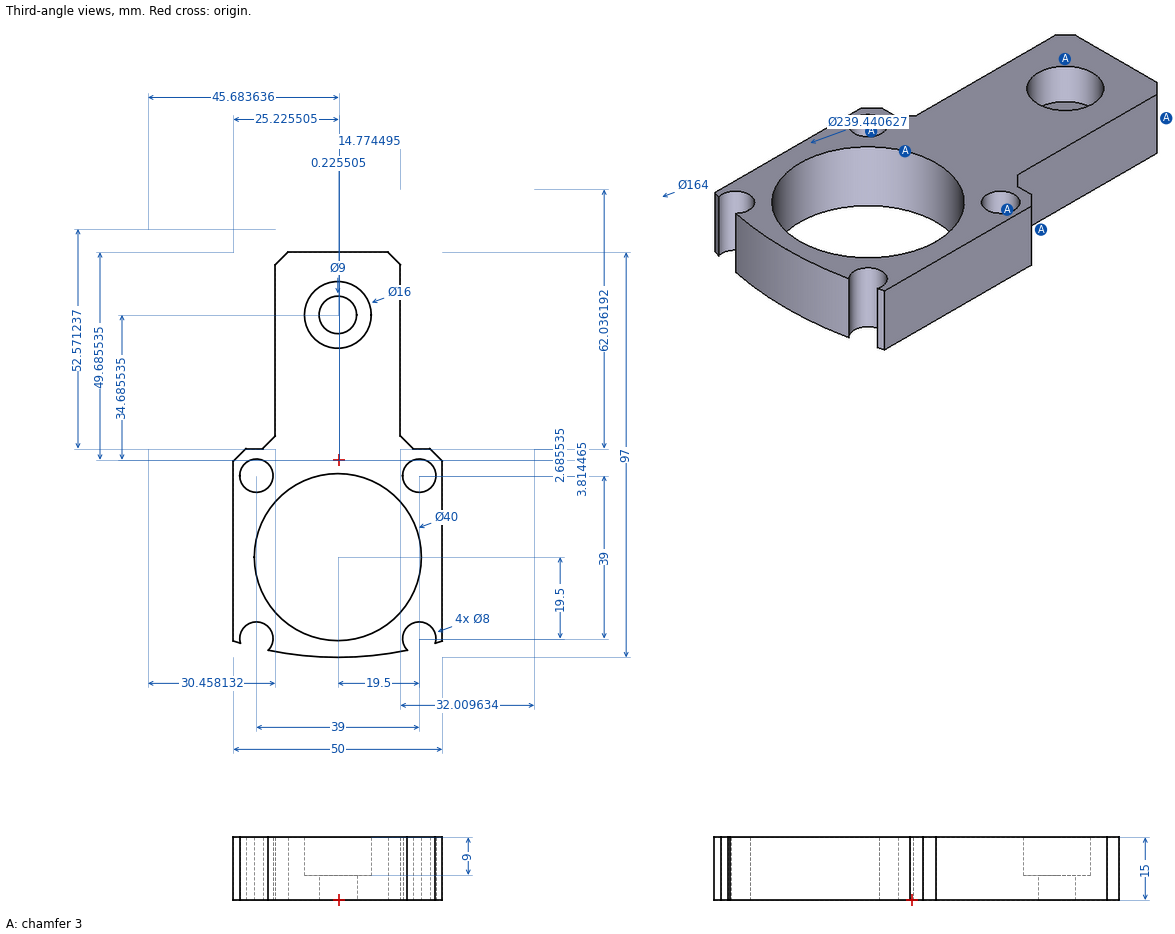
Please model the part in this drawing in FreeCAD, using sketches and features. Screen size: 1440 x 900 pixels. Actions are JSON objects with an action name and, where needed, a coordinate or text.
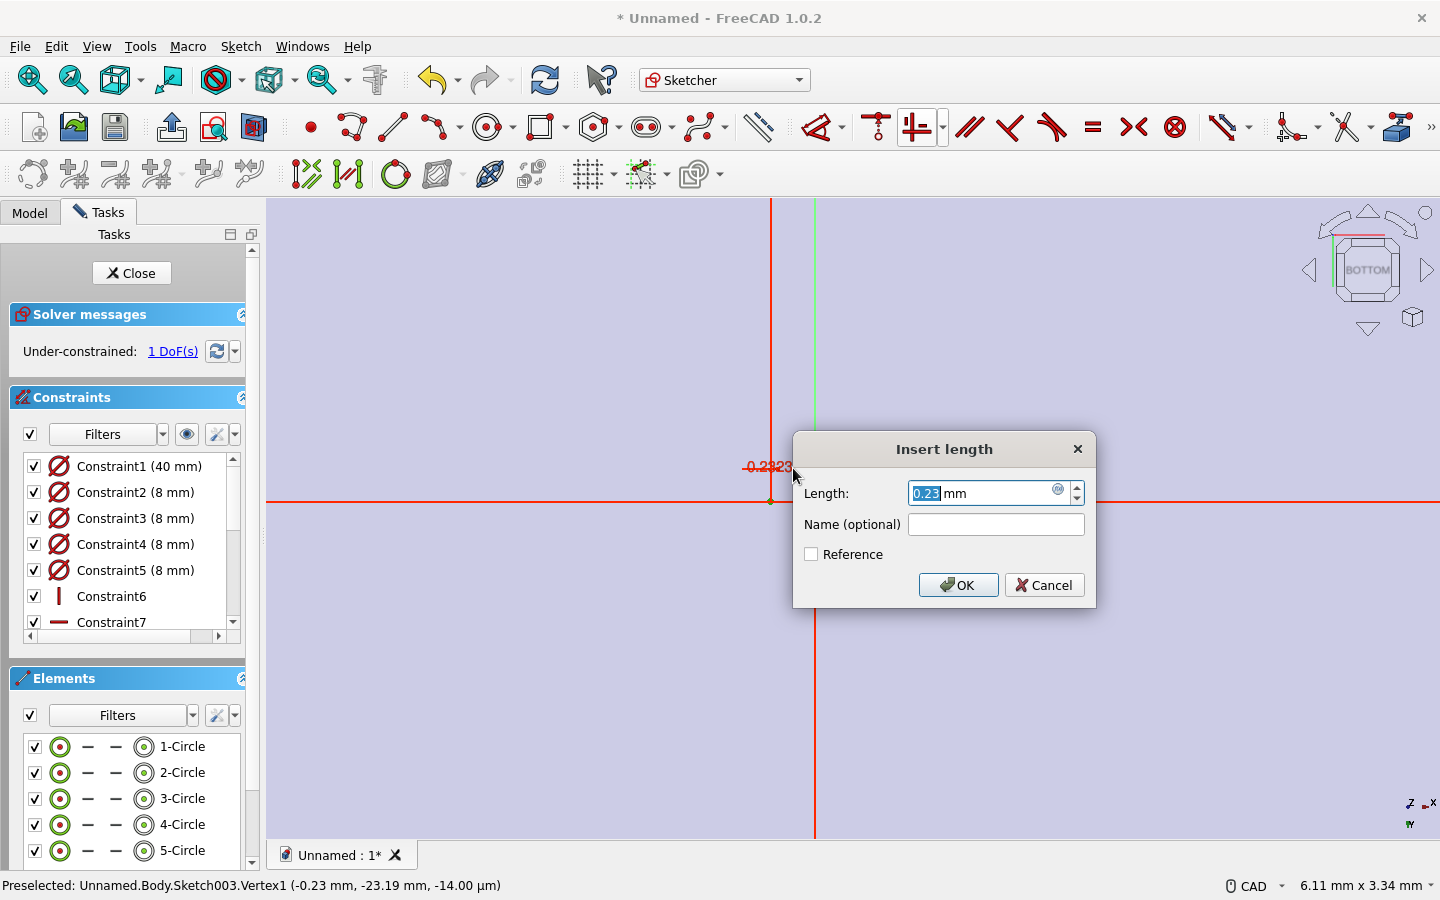
{"action": "type", "text": "0.225505"}
{"action": "key", "text": "Return"}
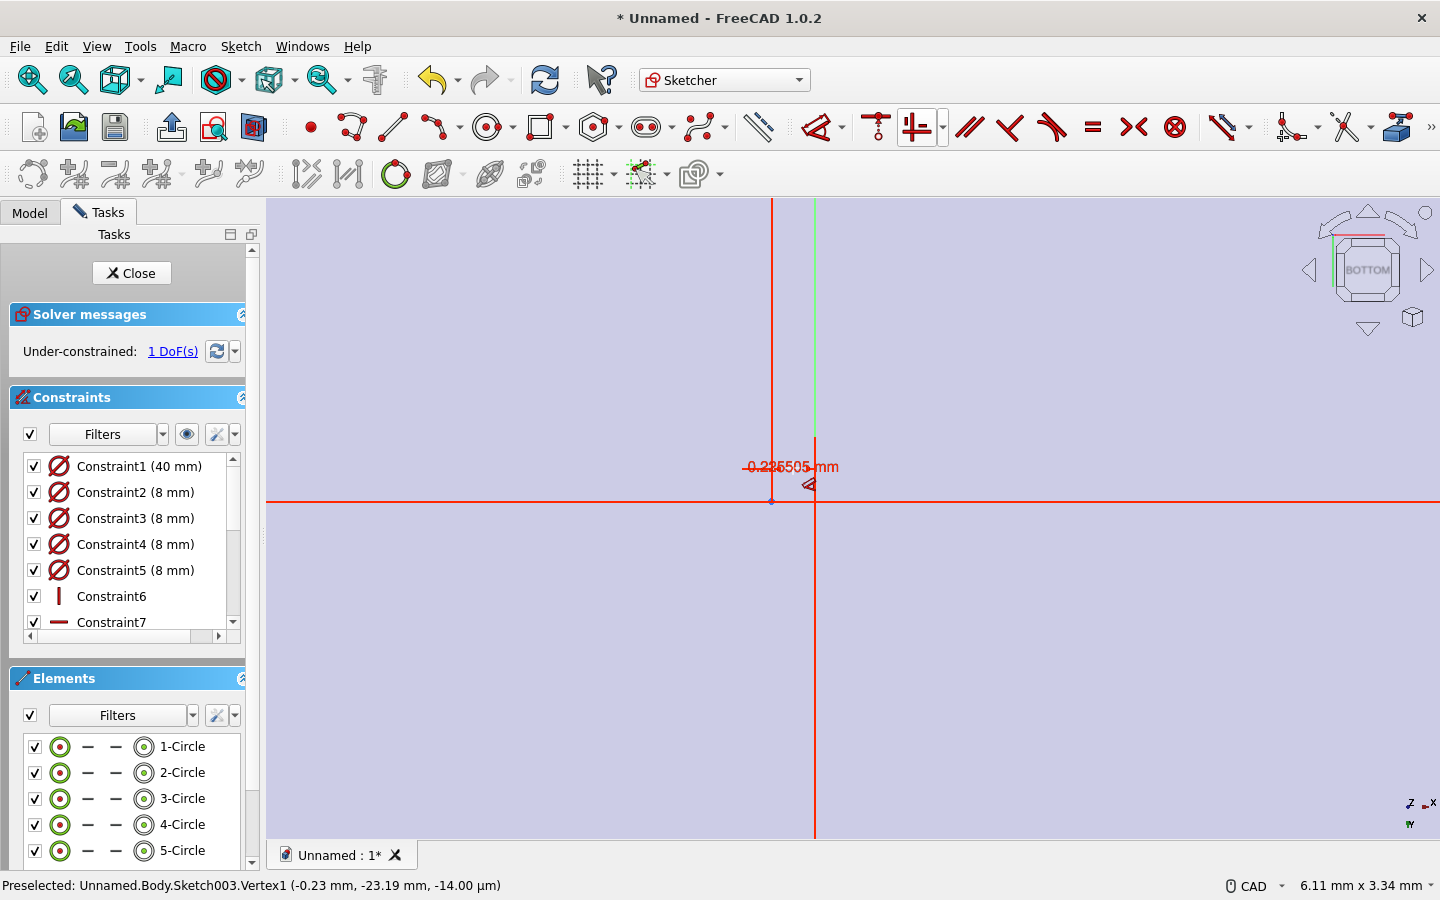
{"action": "scroll", "coordinate": [785, 521], "scroll_direction": "down", "scroll_amount": 15}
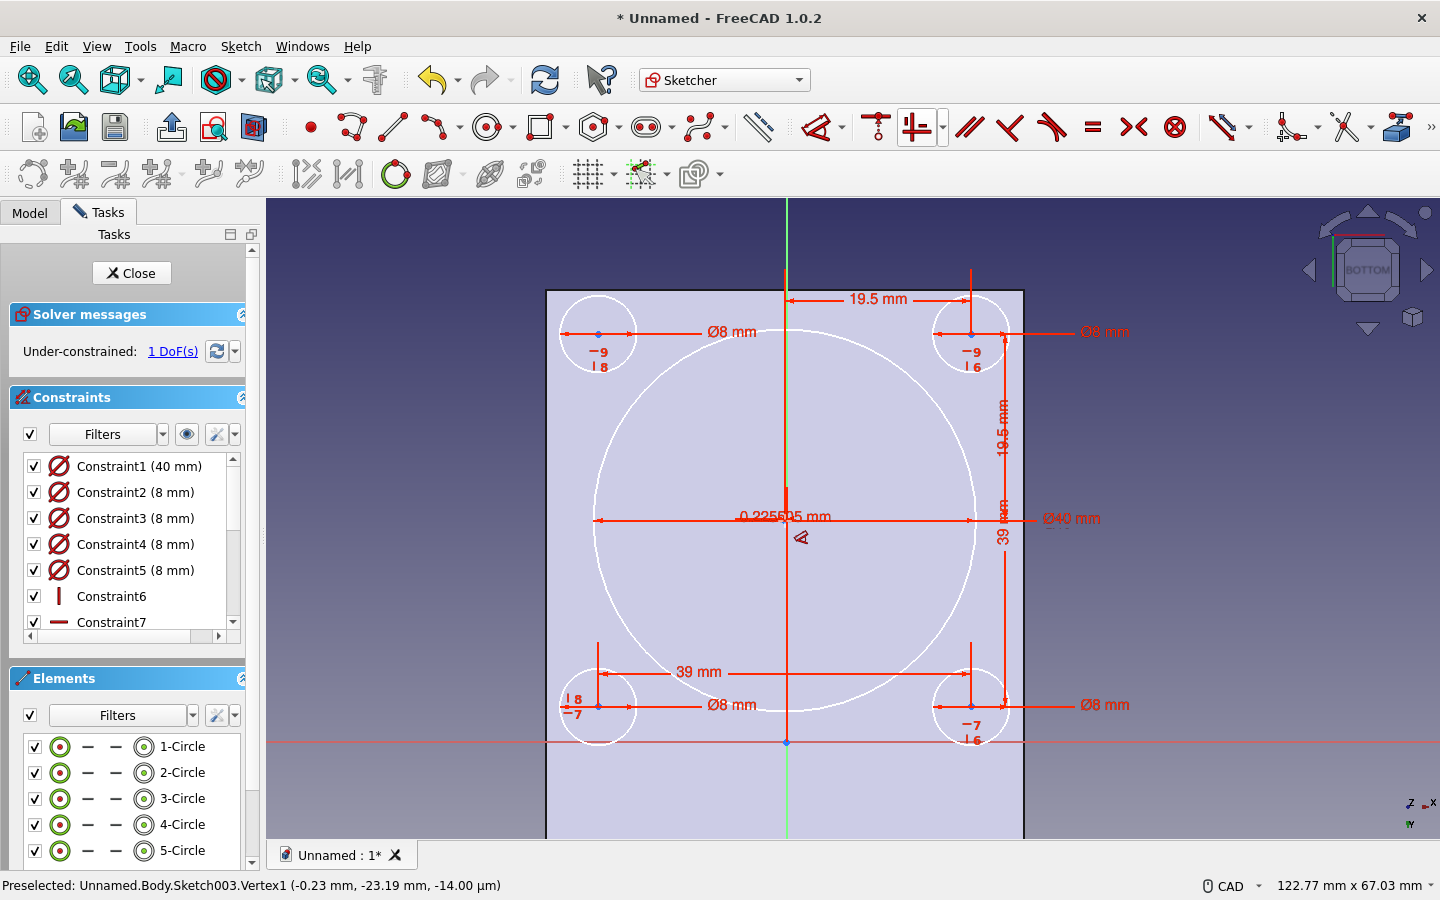
{"action": "left_click", "coordinate": [971, 707]}
{"action": "left_click", "coordinate": [753, 725]}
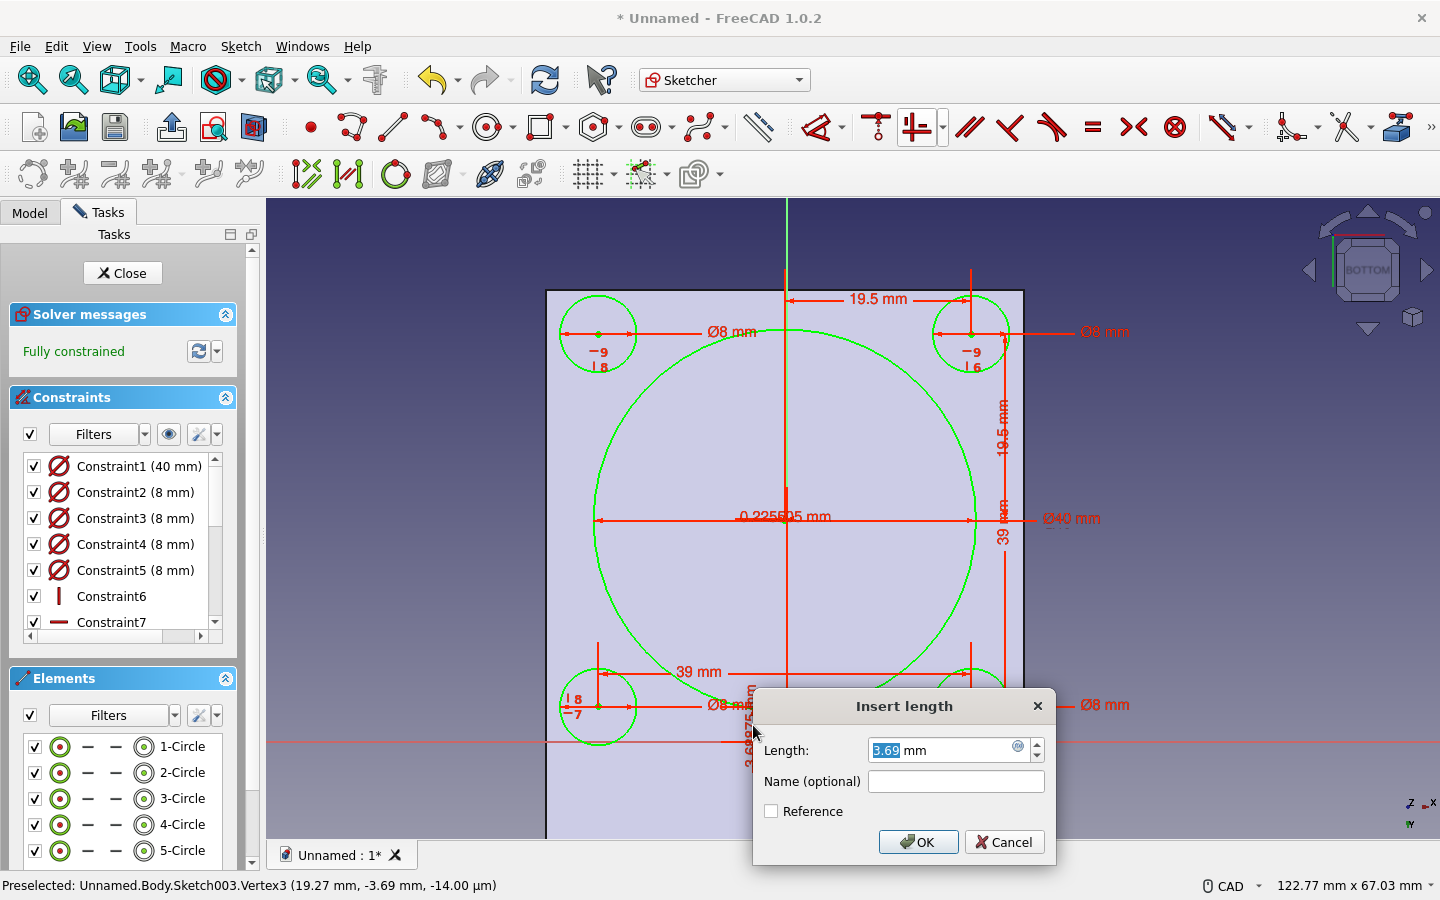
{"action": "type", "text": "3.814465"}
{"action": "key", "text": "Return"}
{"action": "key", "text": "Escape"}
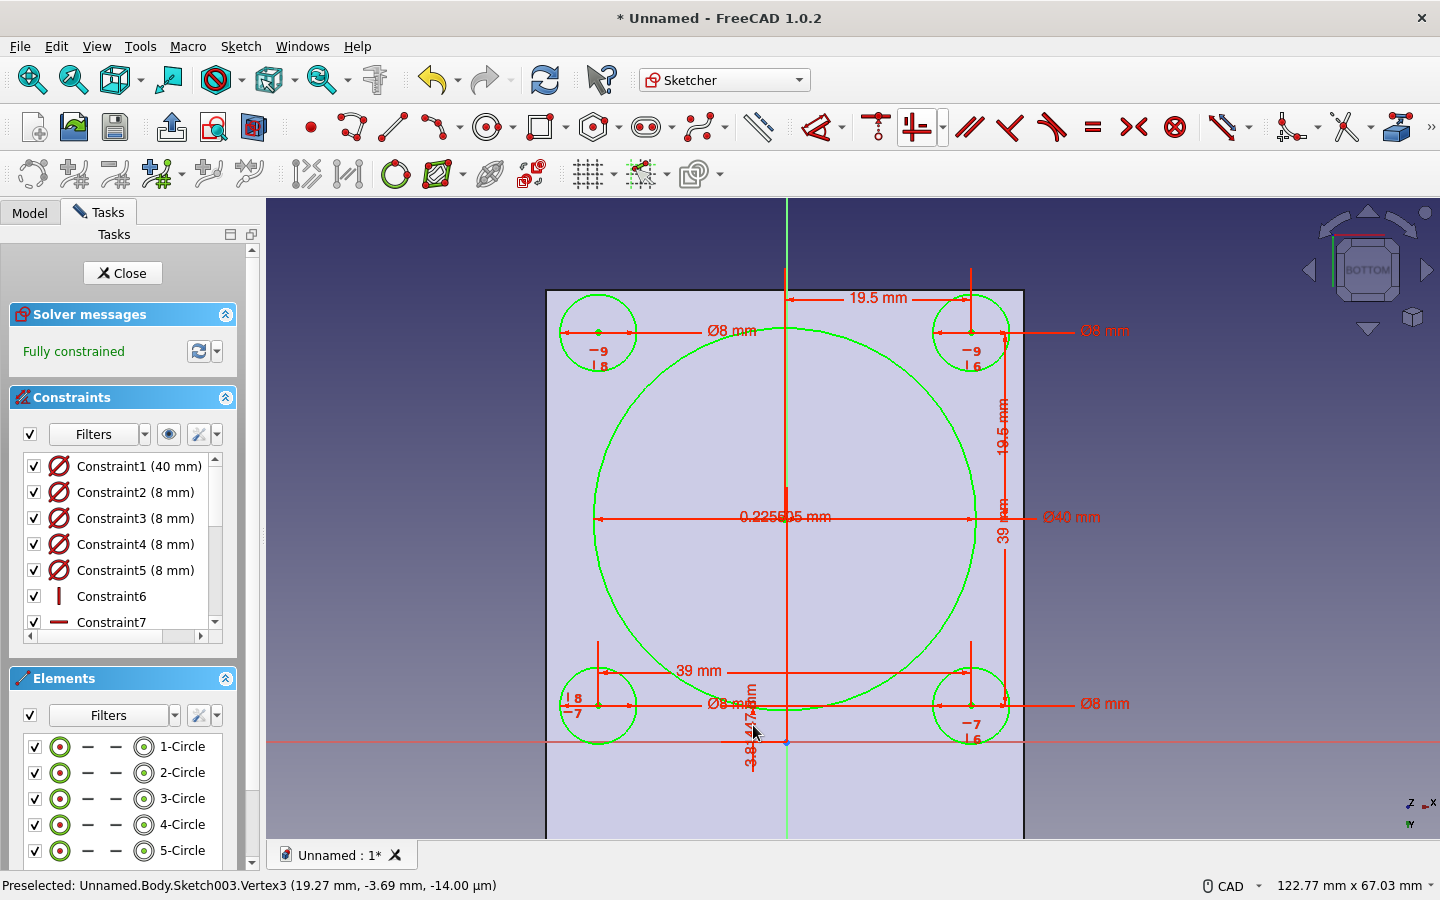
{"action": "left_click", "coordinate": [123, 273]}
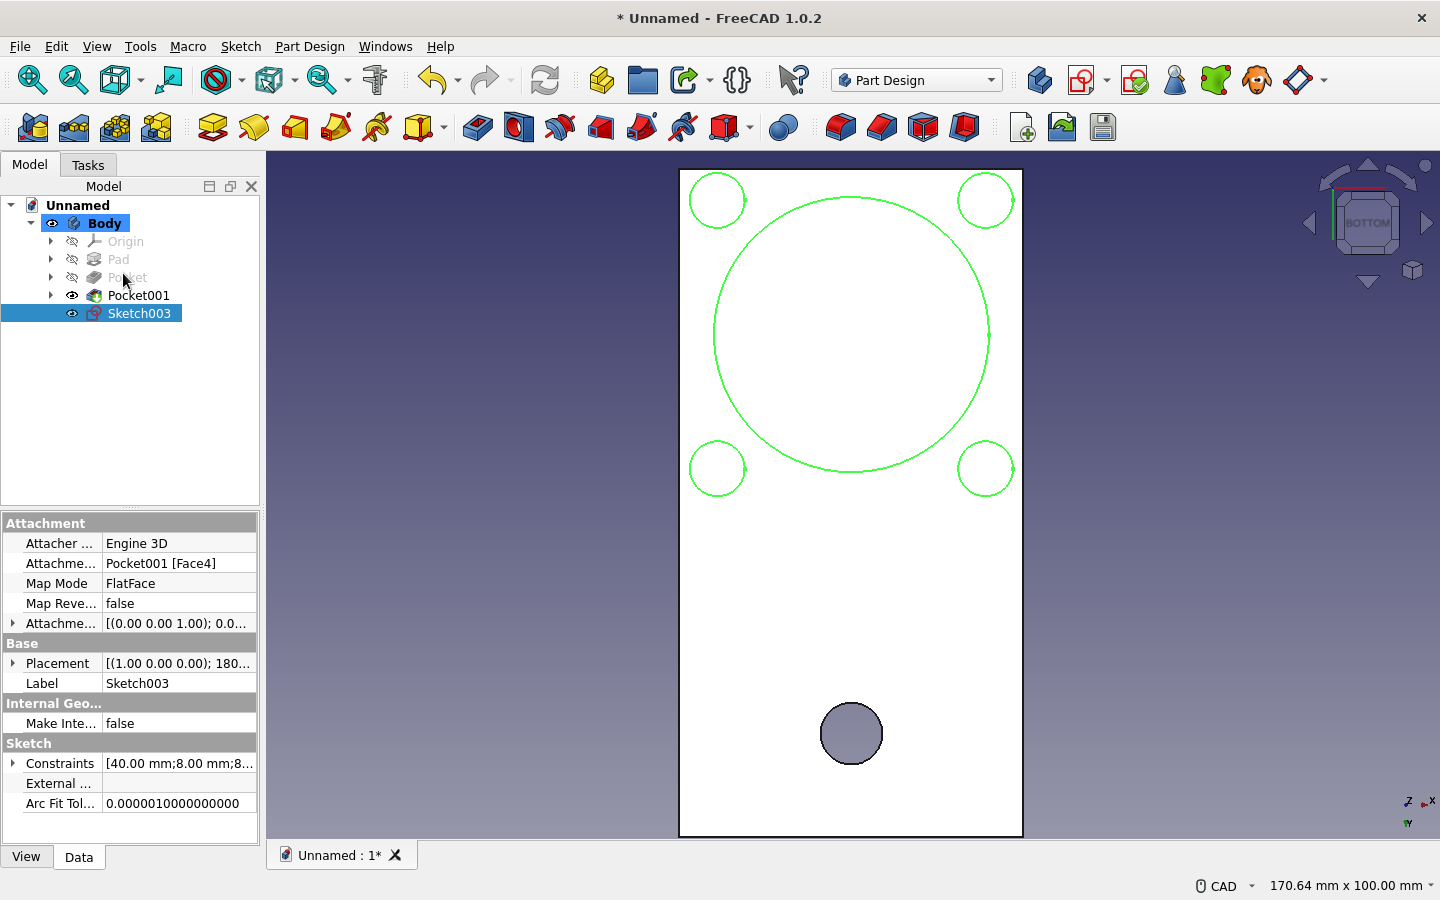
{"action": "left_click", "coordinate": [478, 128]}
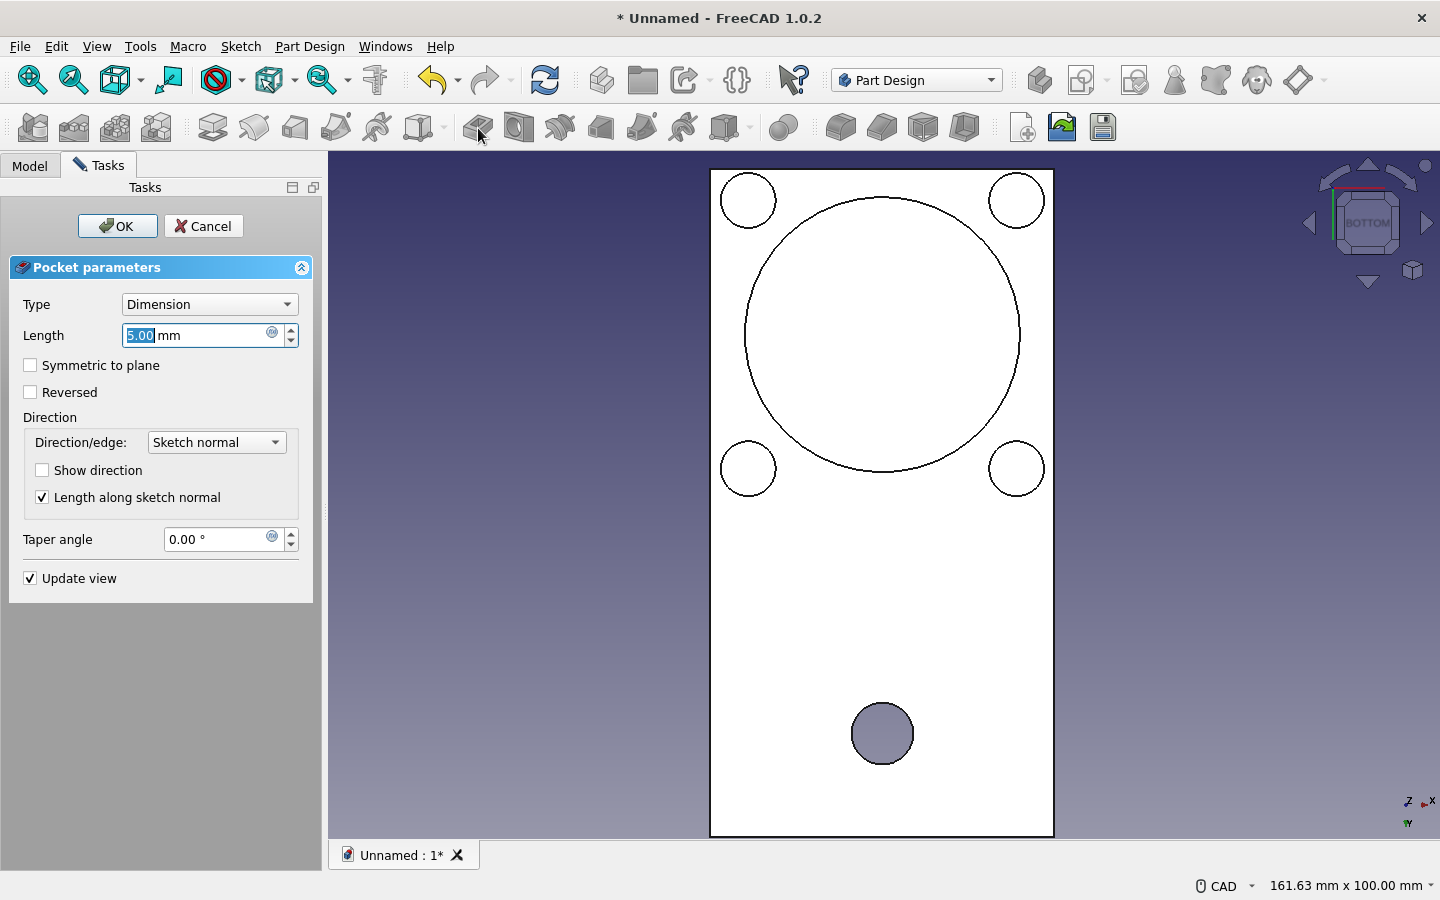
{"action": "left_click", "coordinate": [210, 304]}